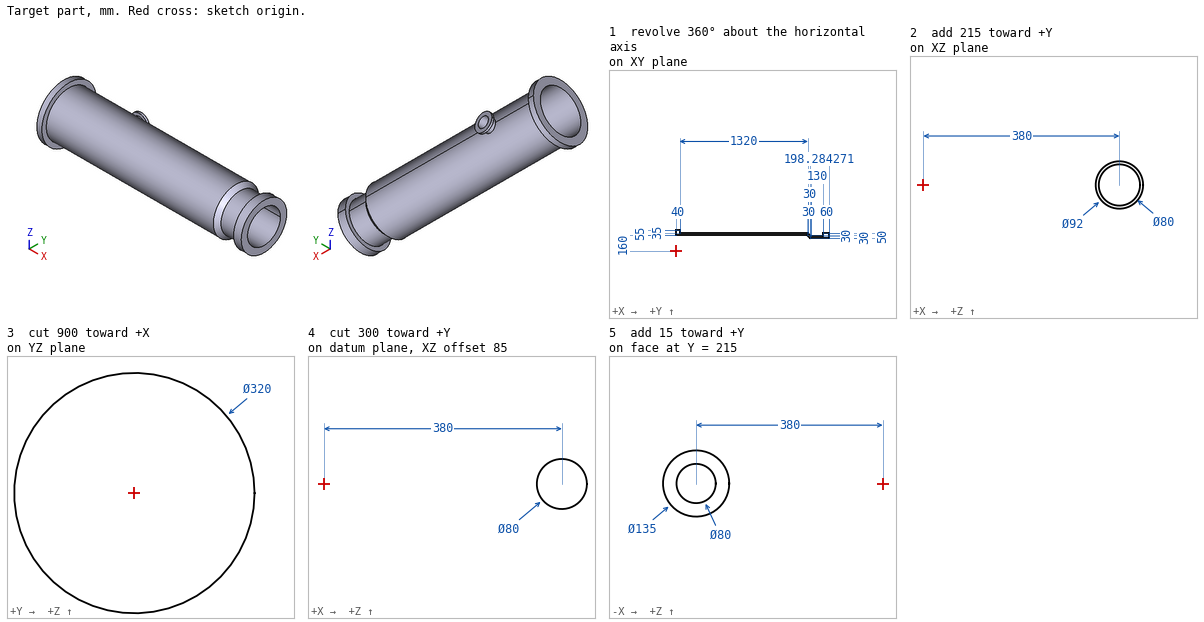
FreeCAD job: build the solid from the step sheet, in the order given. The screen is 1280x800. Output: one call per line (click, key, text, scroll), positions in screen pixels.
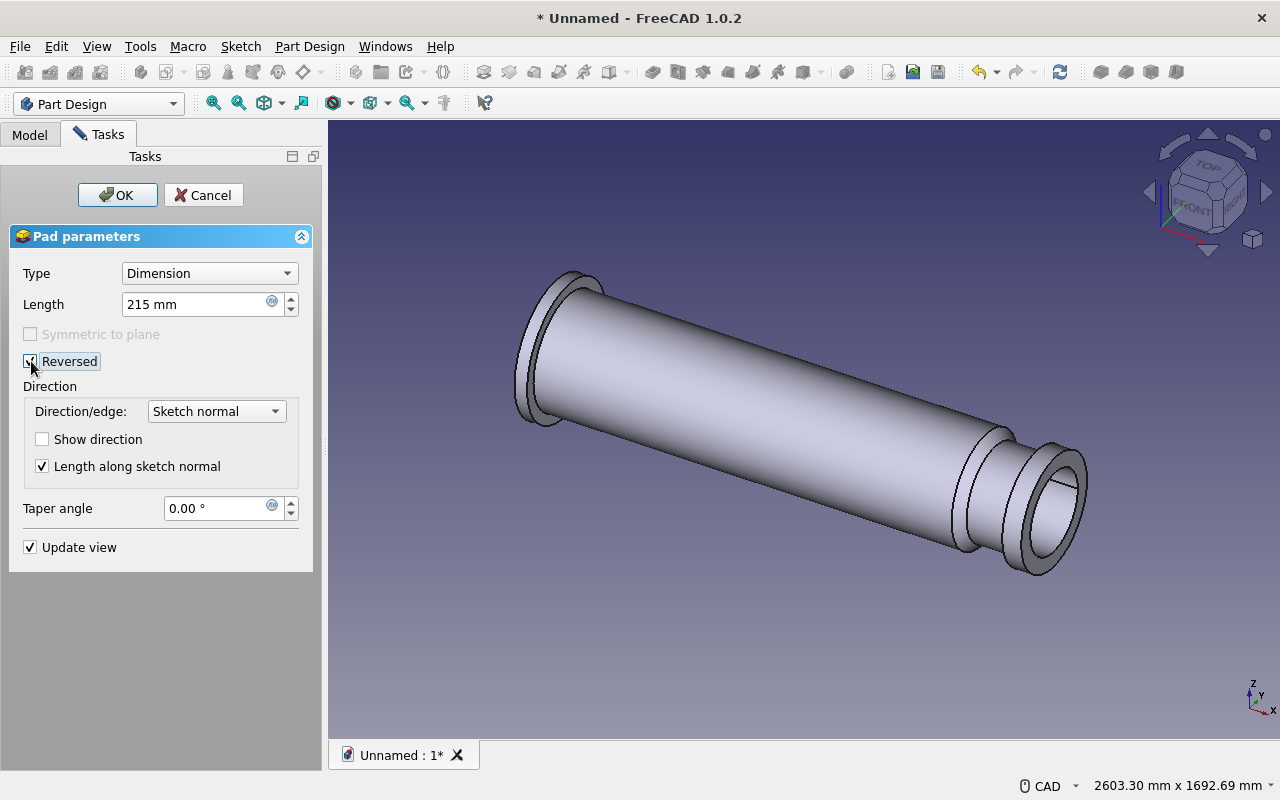
click(118, 195)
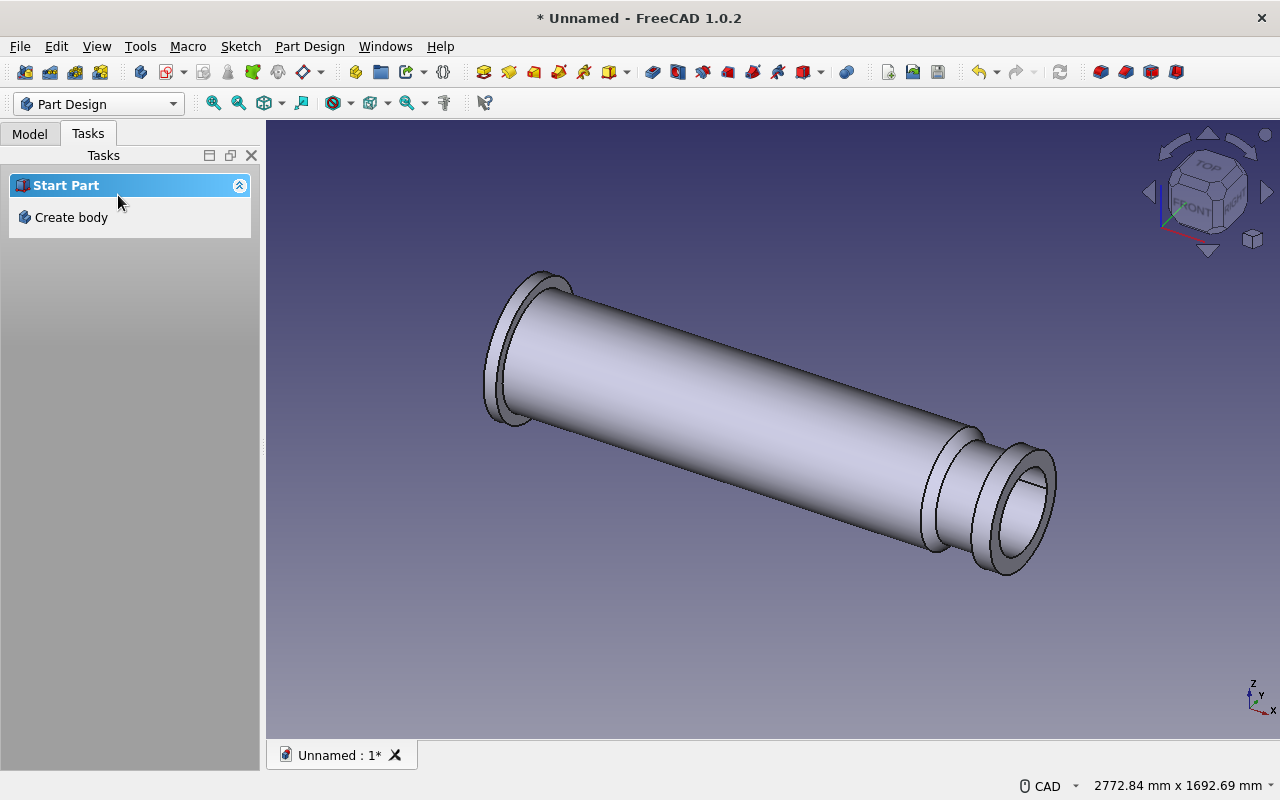
click(166, 72)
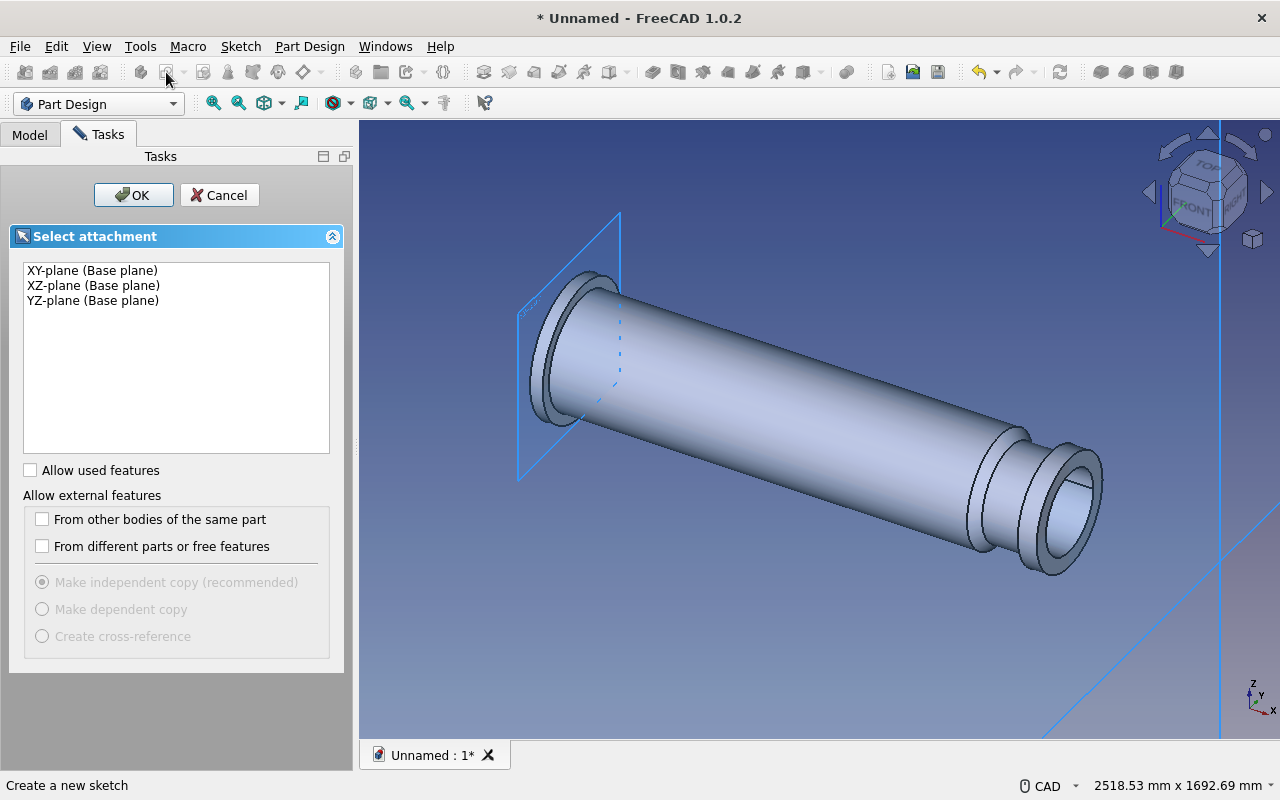
click(84, 300)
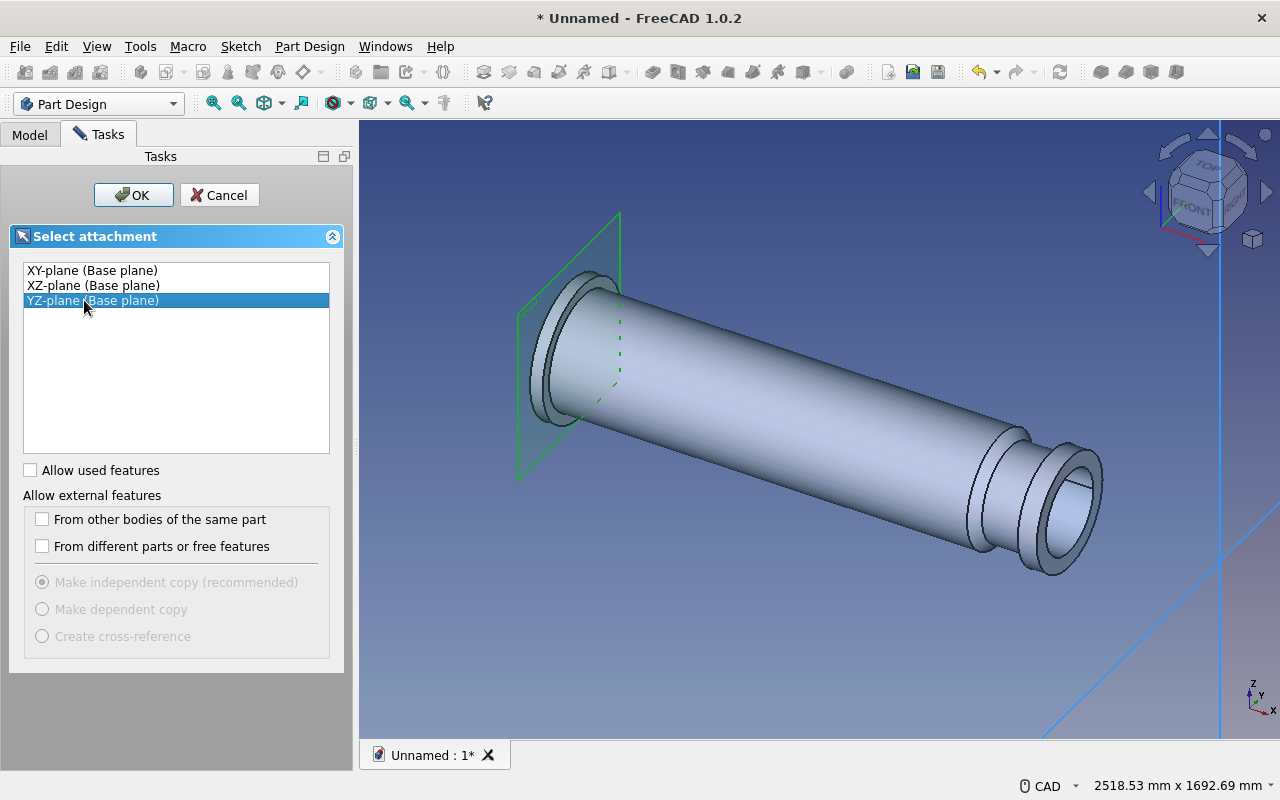
click(134, 195)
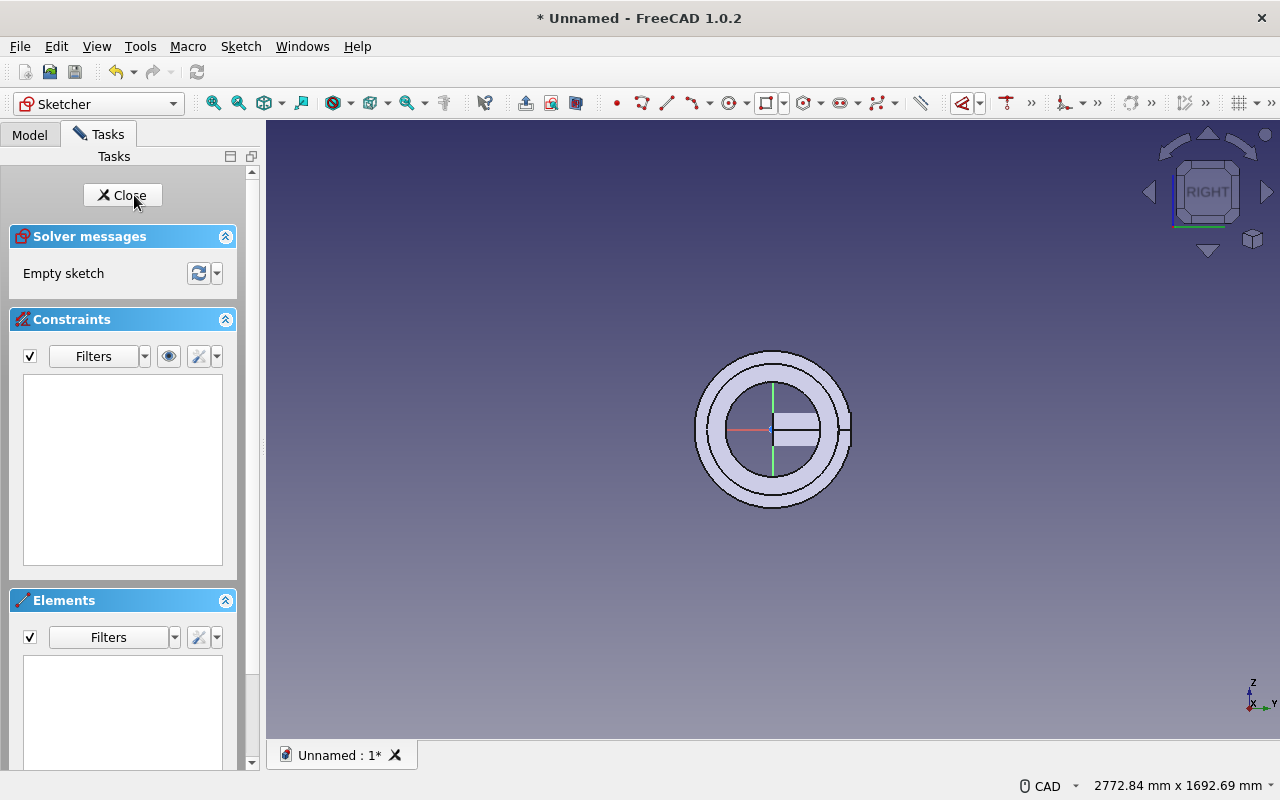
click(576, 104)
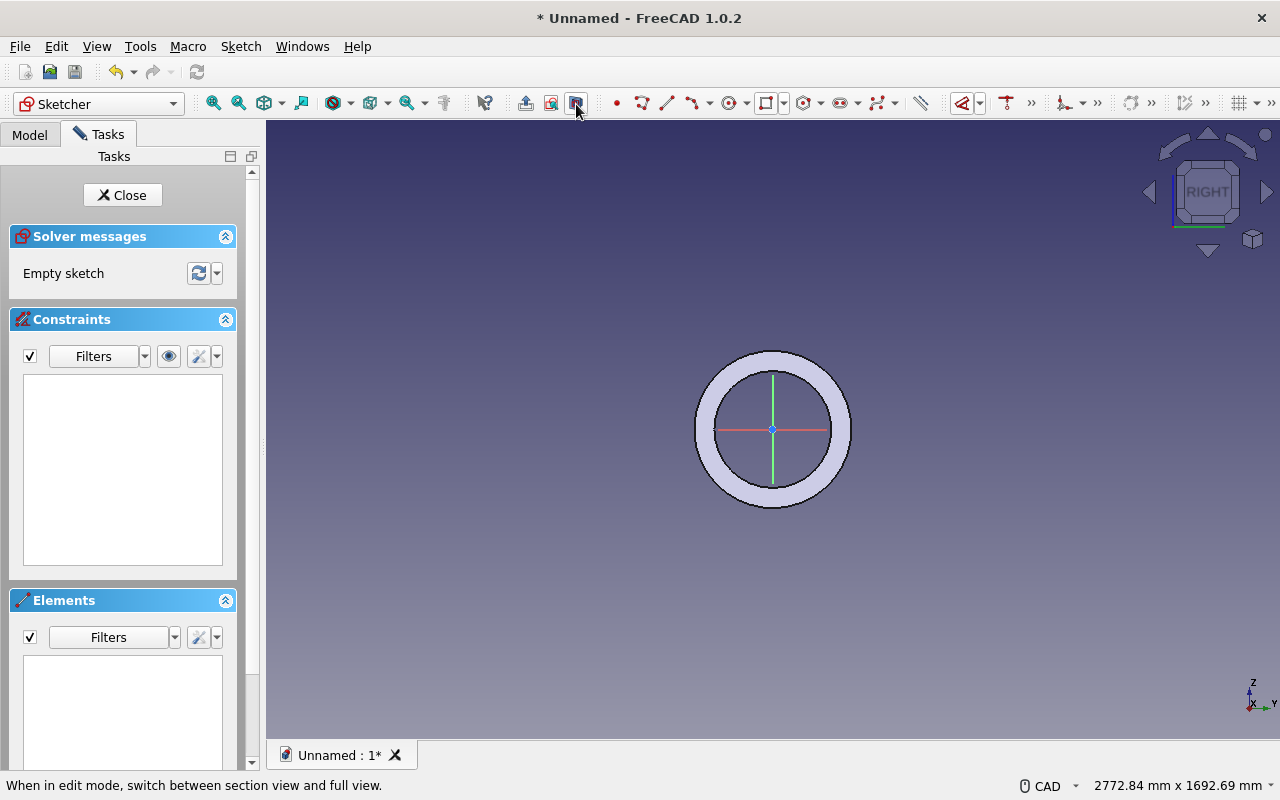
scroll(802, 430, up, 6)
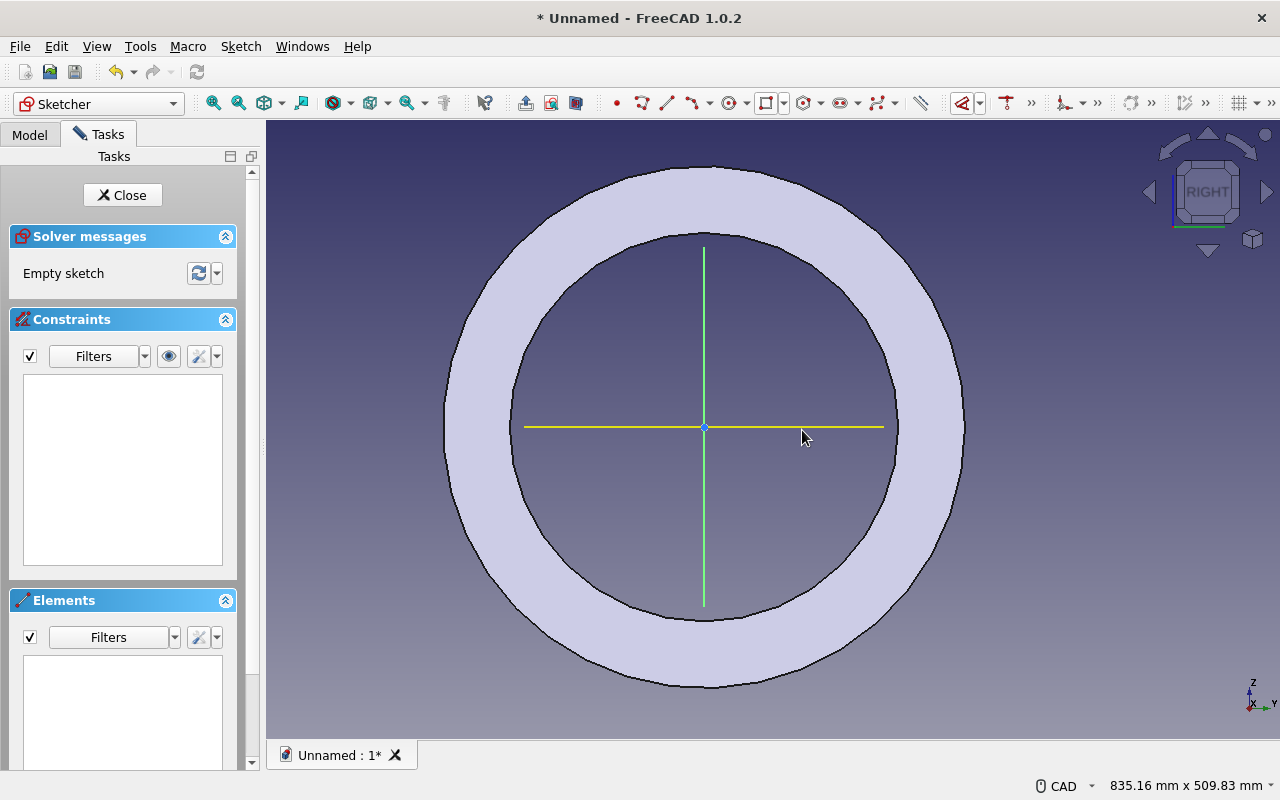
key(g)
key(c)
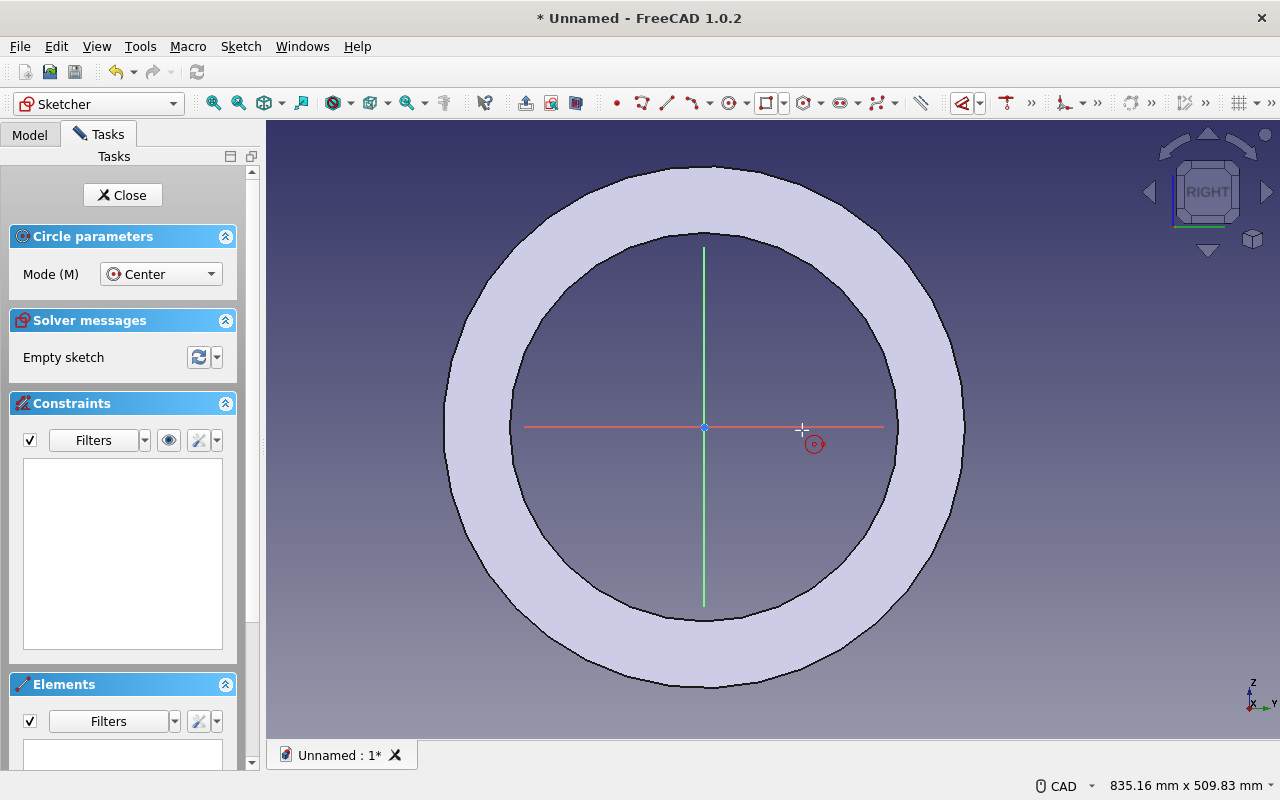
click(704, 427)
move(841, 290)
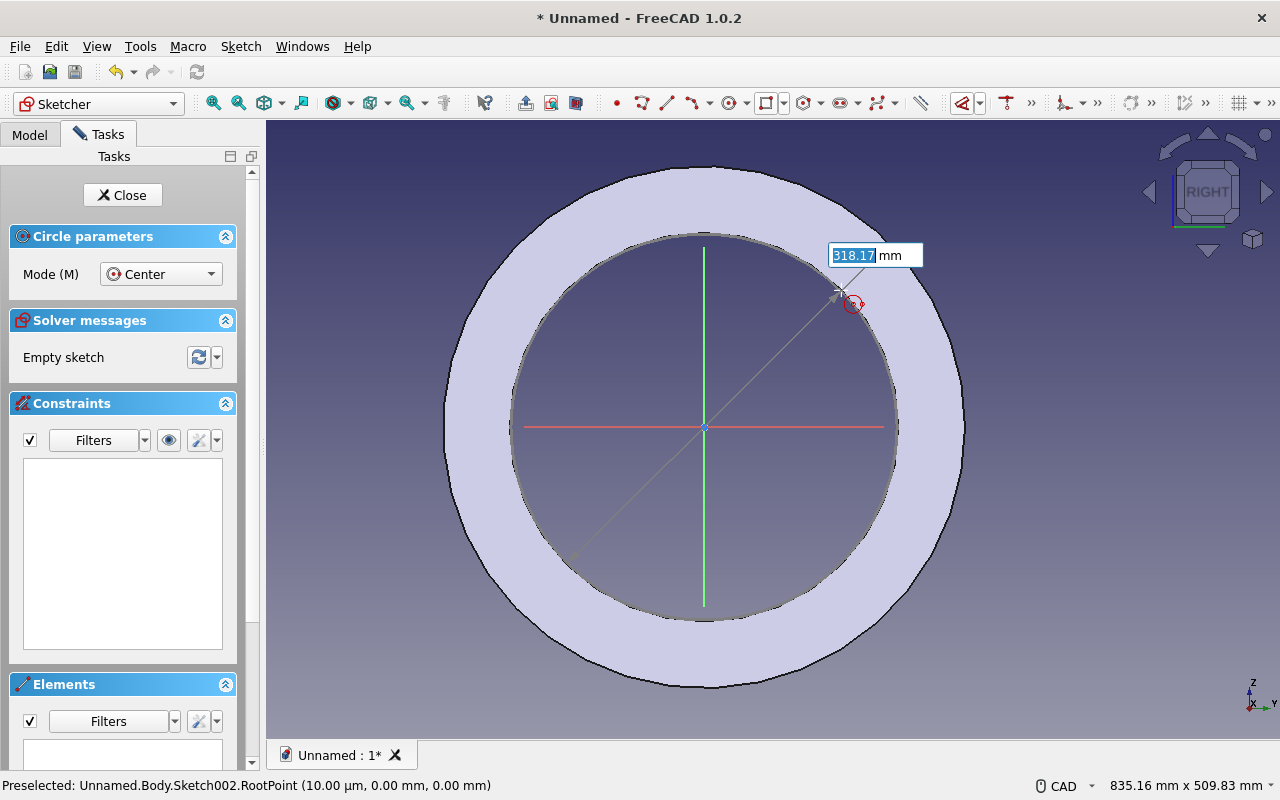
text(320)
key(Return)
key(Escape)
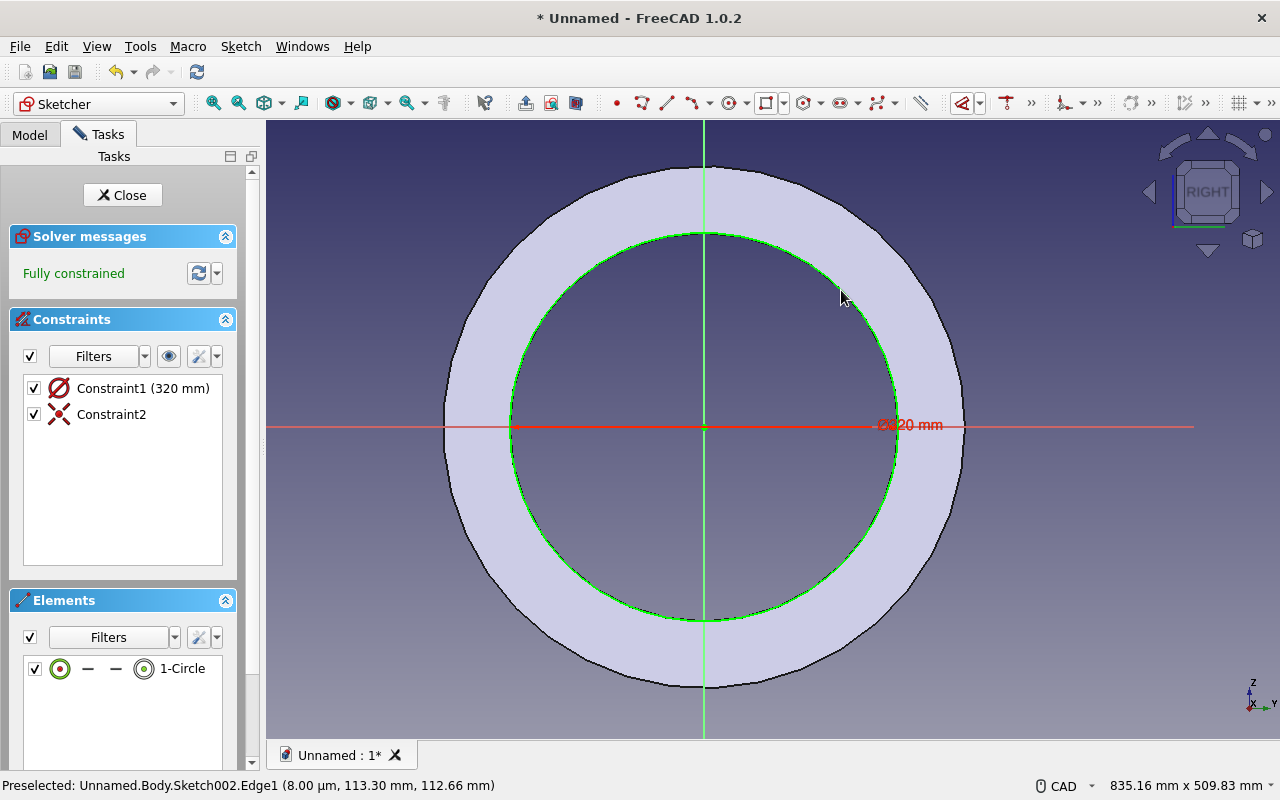
click(123, 195)